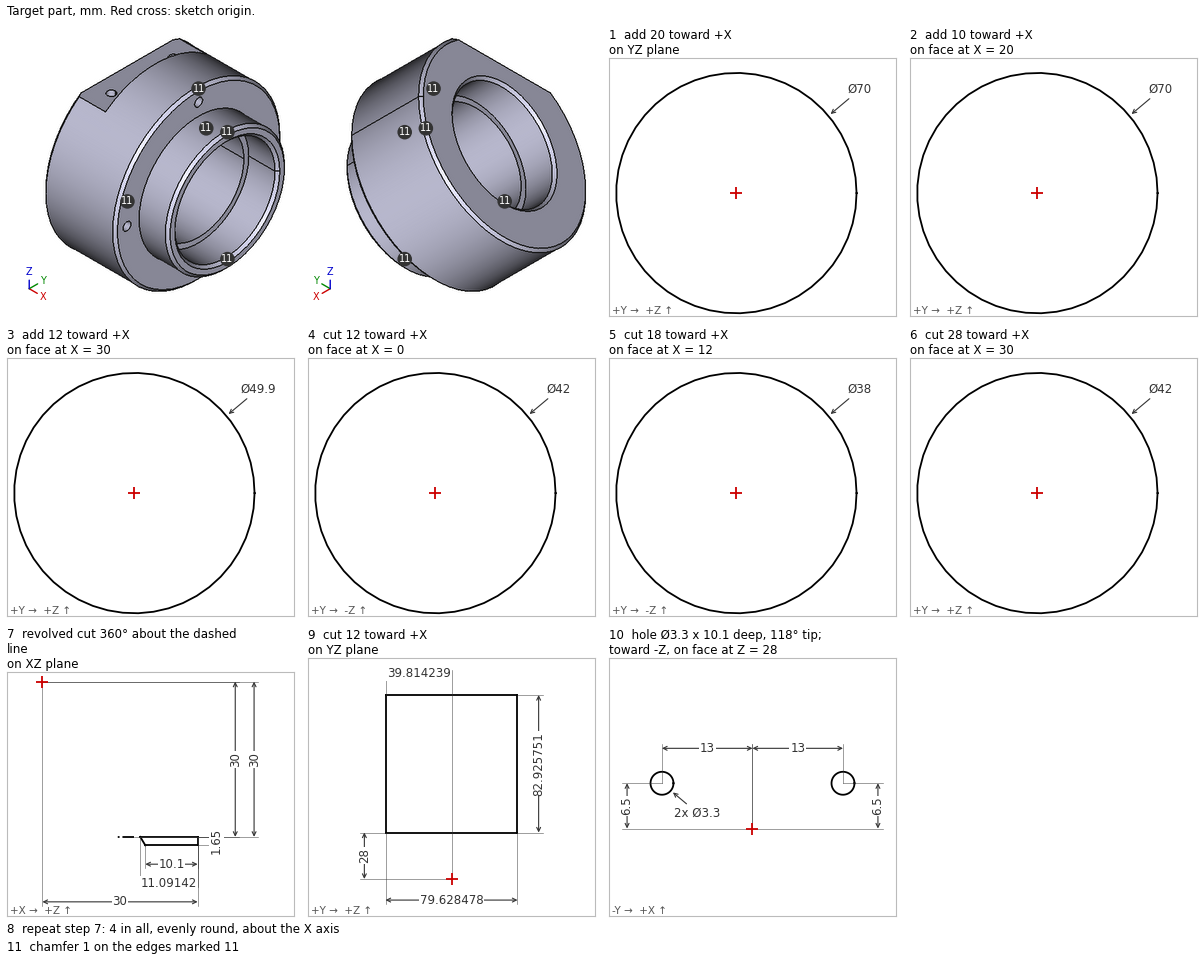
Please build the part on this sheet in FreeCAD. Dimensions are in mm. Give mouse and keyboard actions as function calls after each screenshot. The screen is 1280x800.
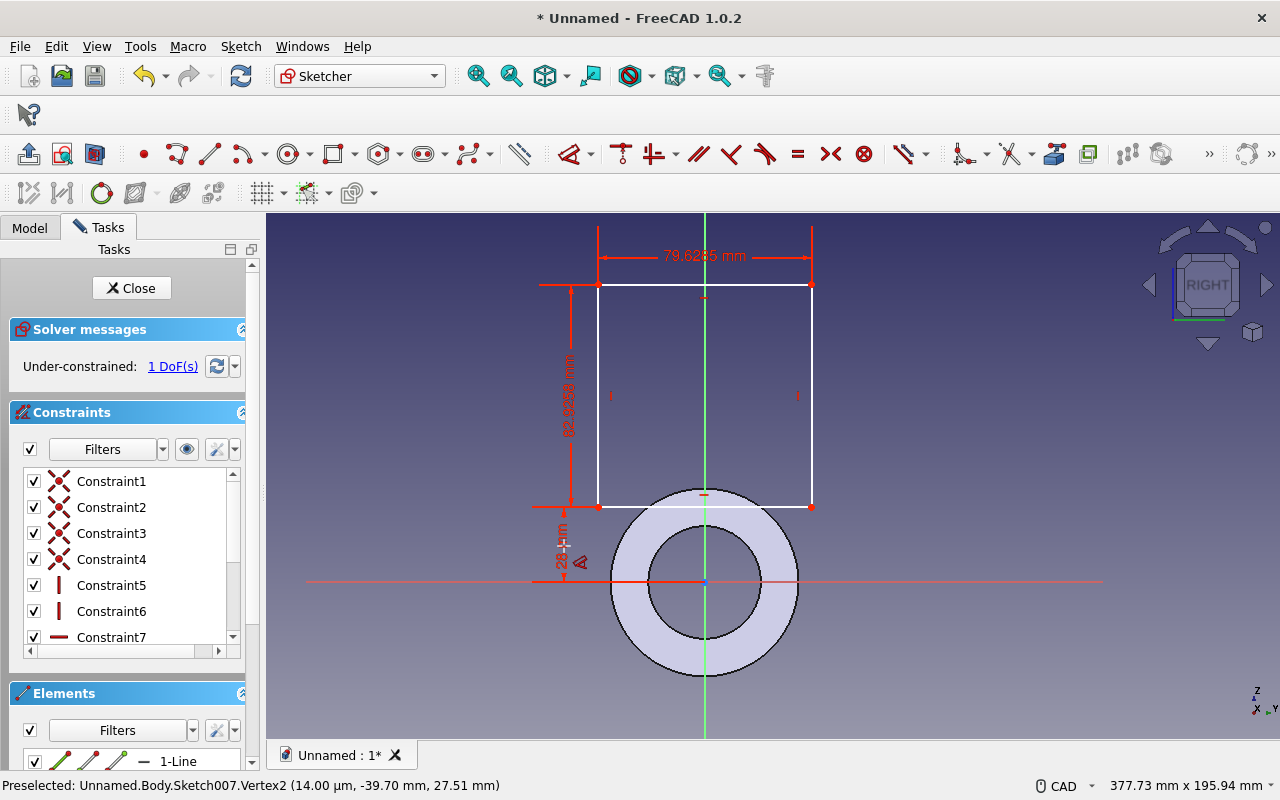
click(598, 285)
click(651, 251)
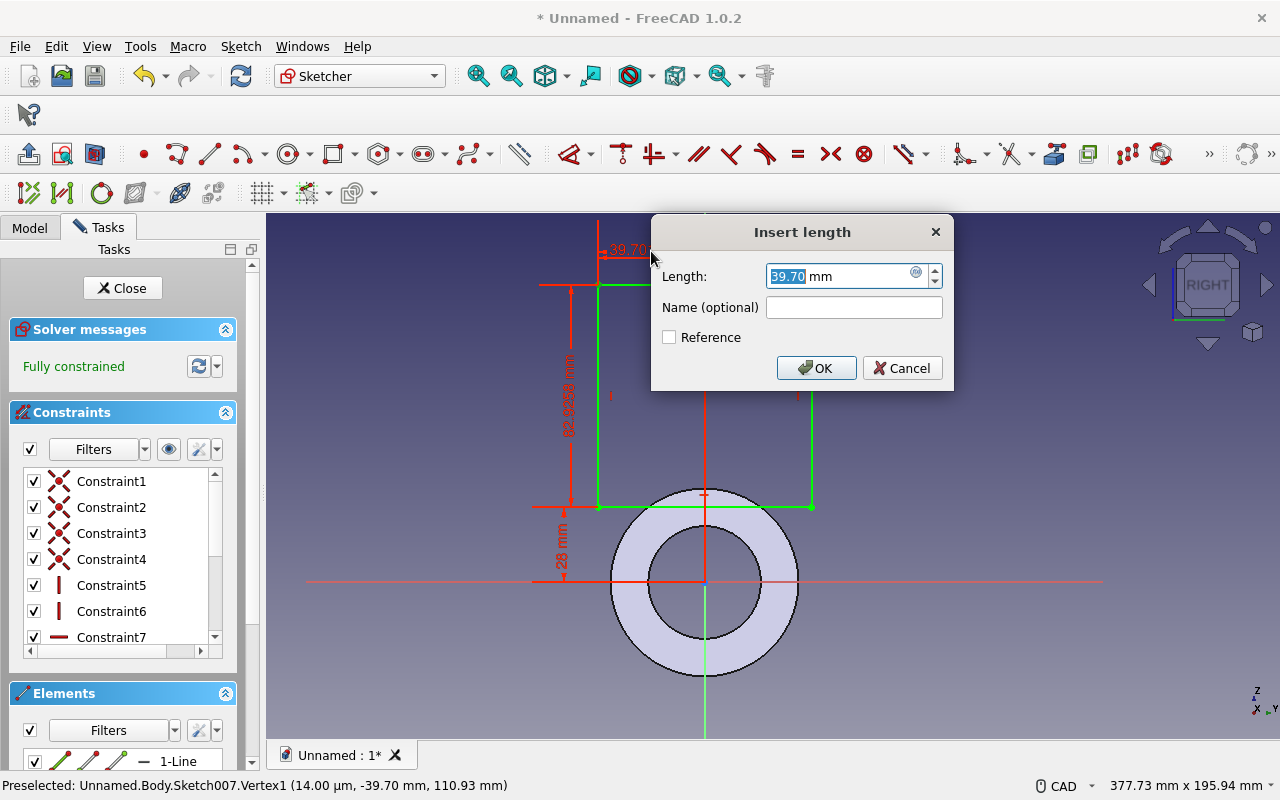
text(39.814239)
key(Return)
key(Escape)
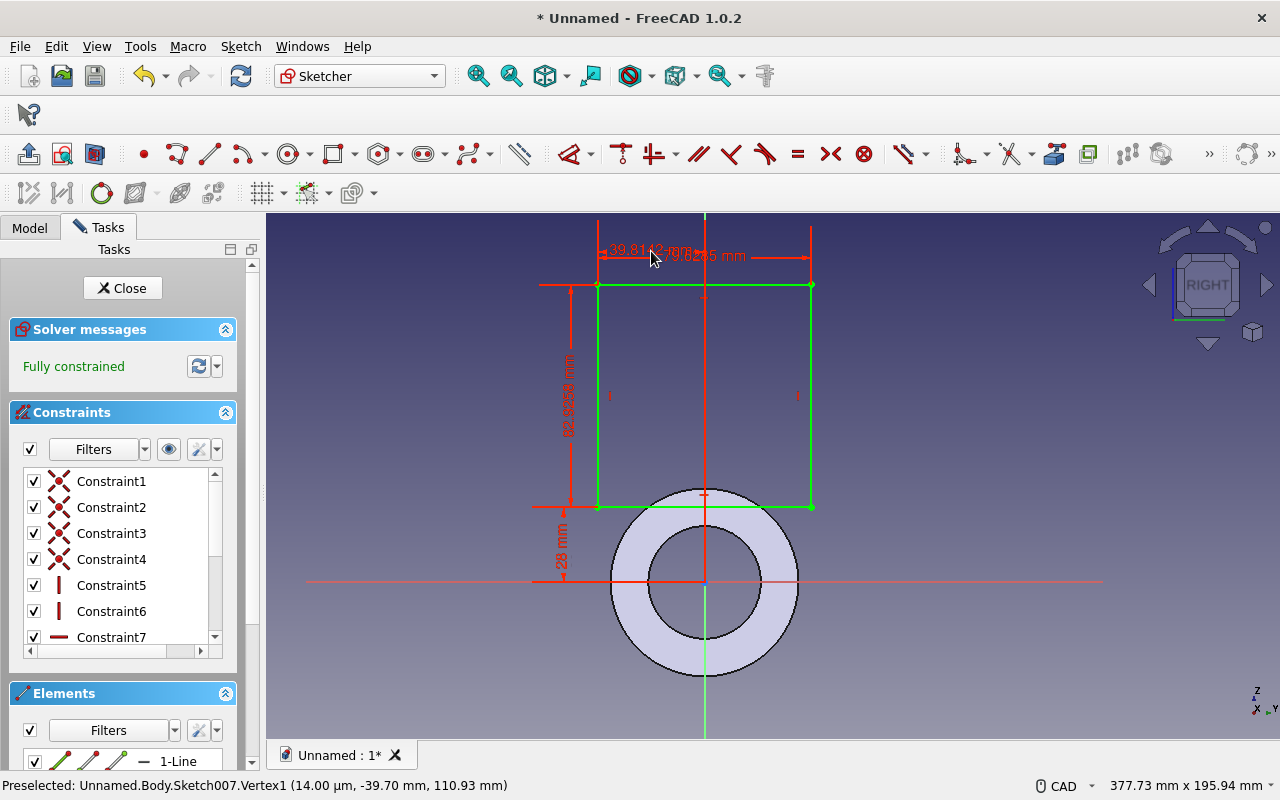
click(123, 288)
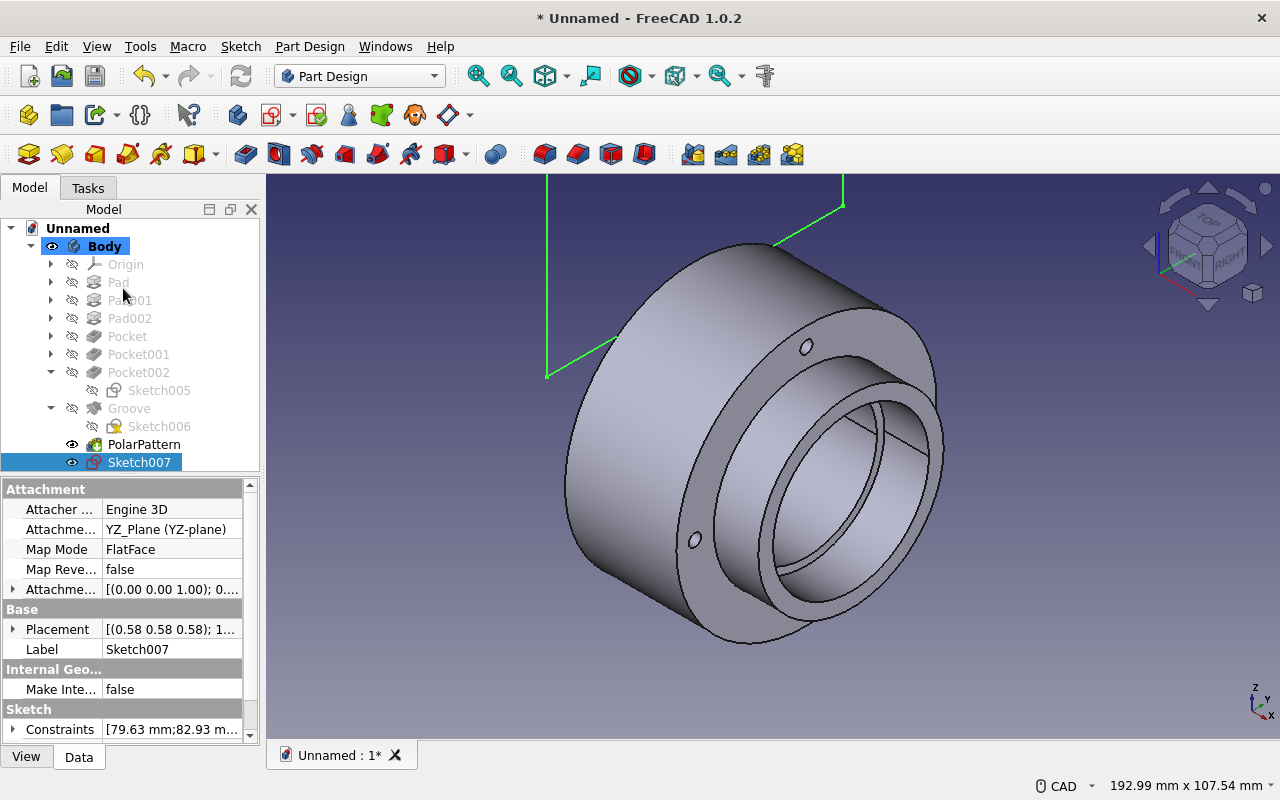
click(246, 154)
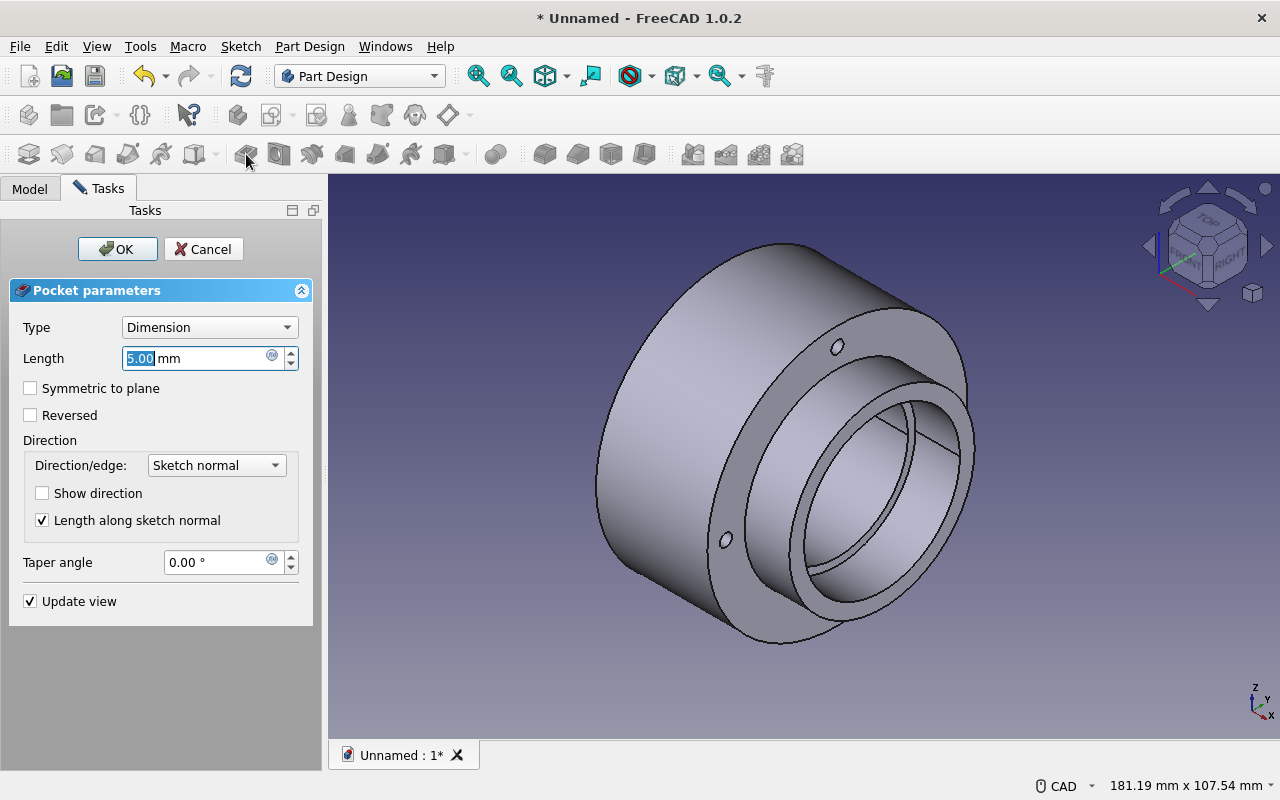
text(12)
key(Tab)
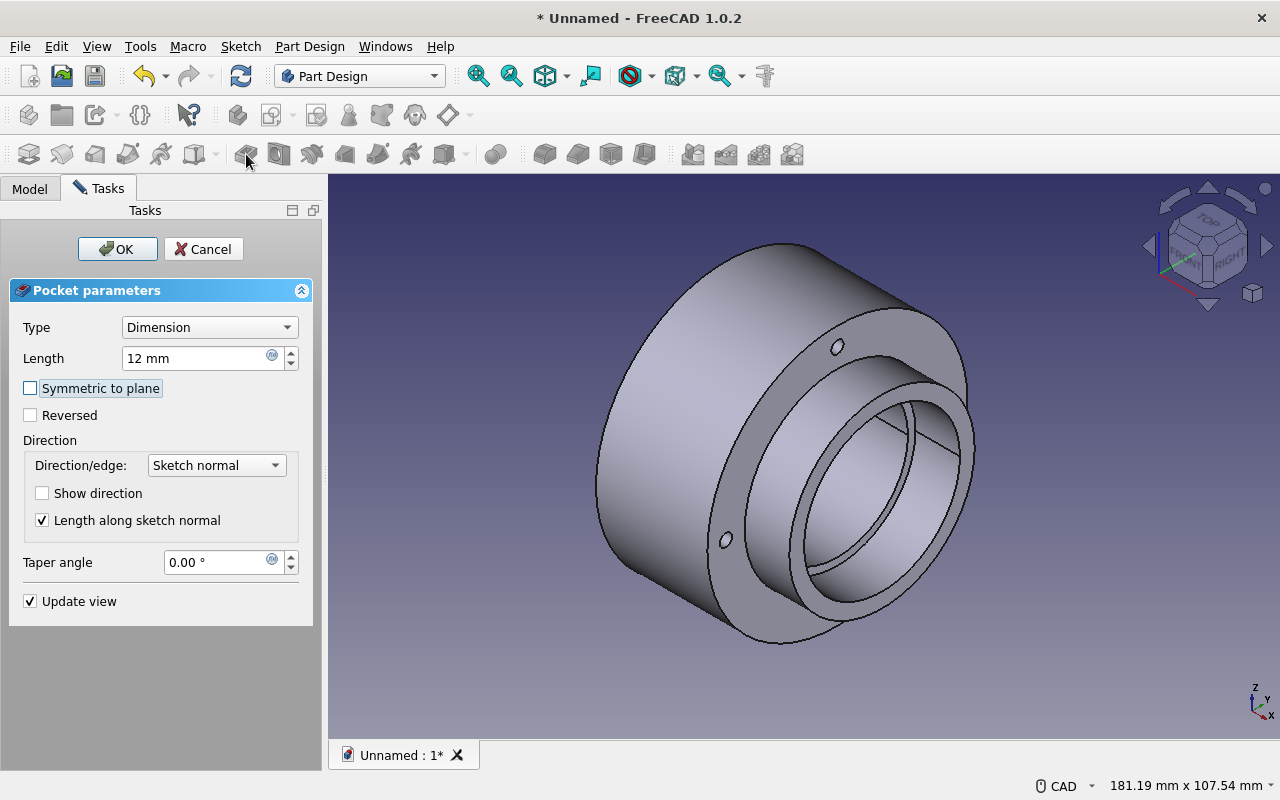
click(31, 415)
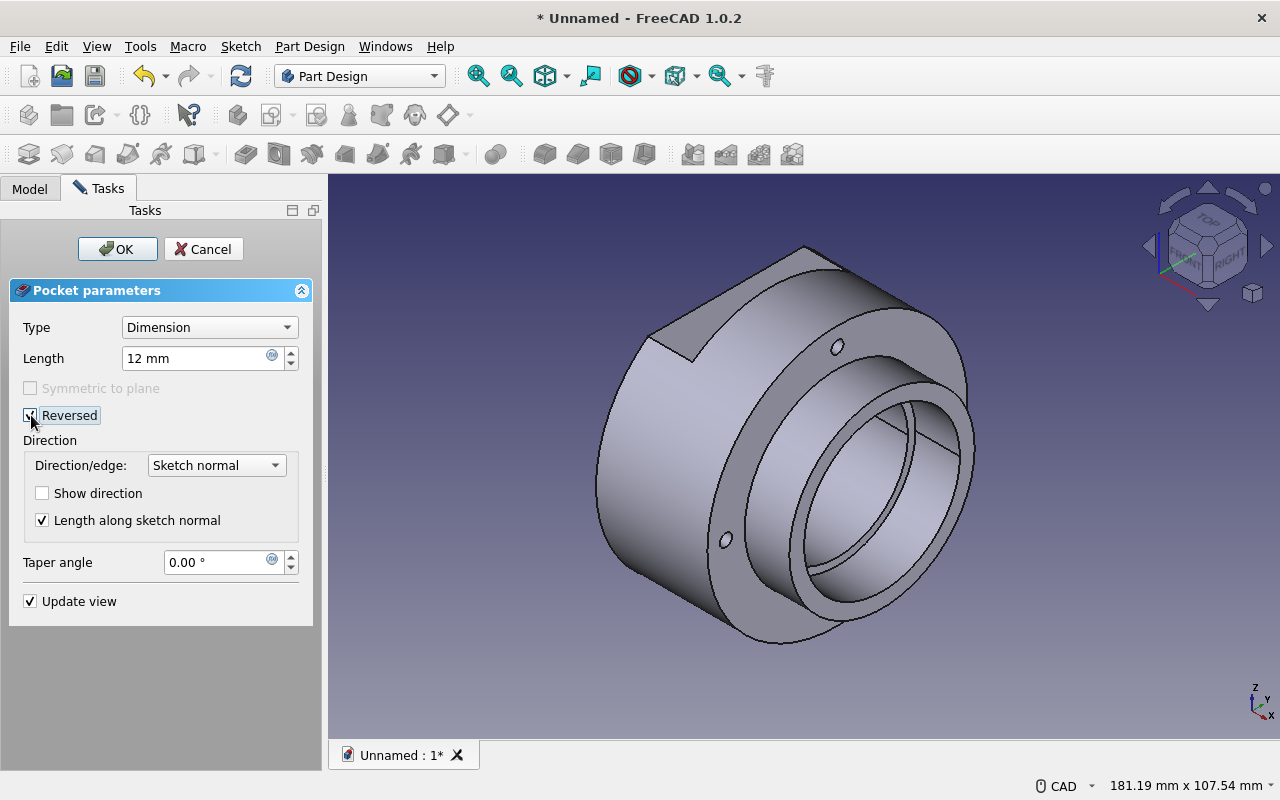
click(118, 249)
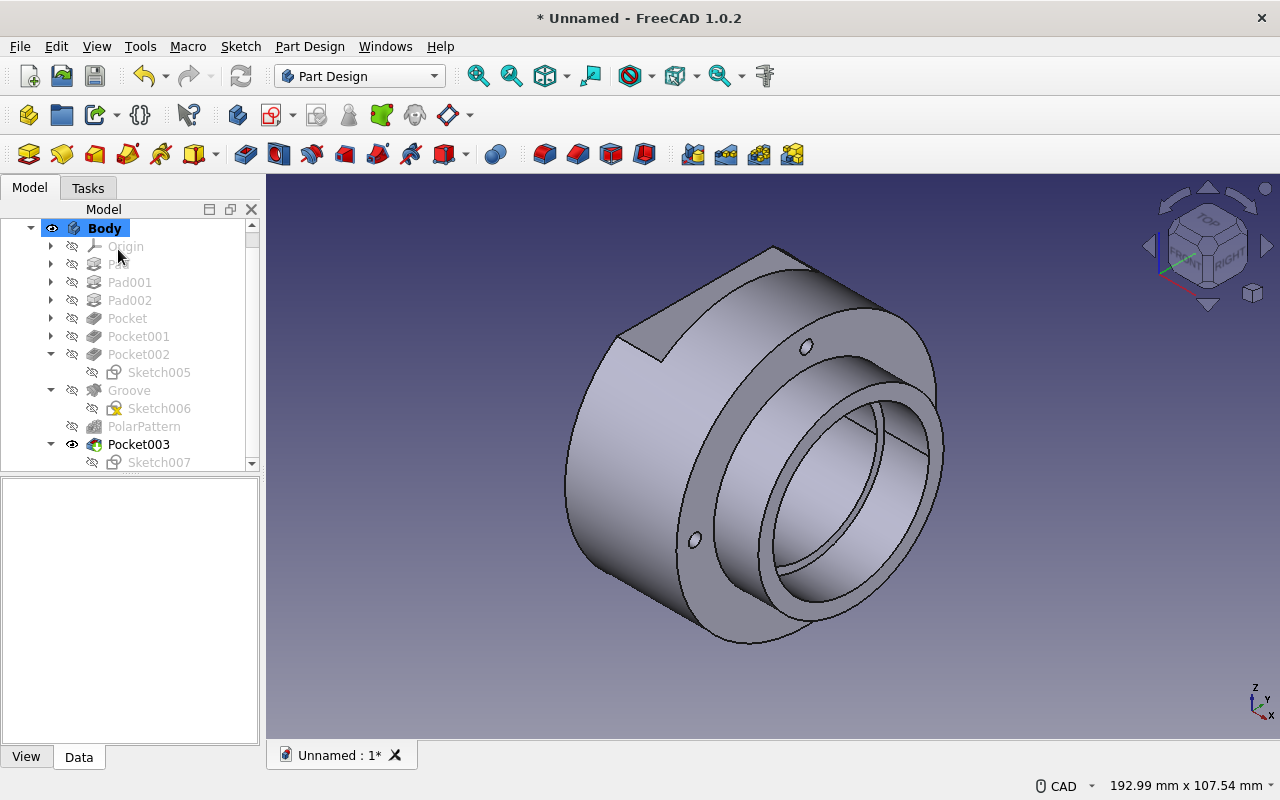
click(673, 329)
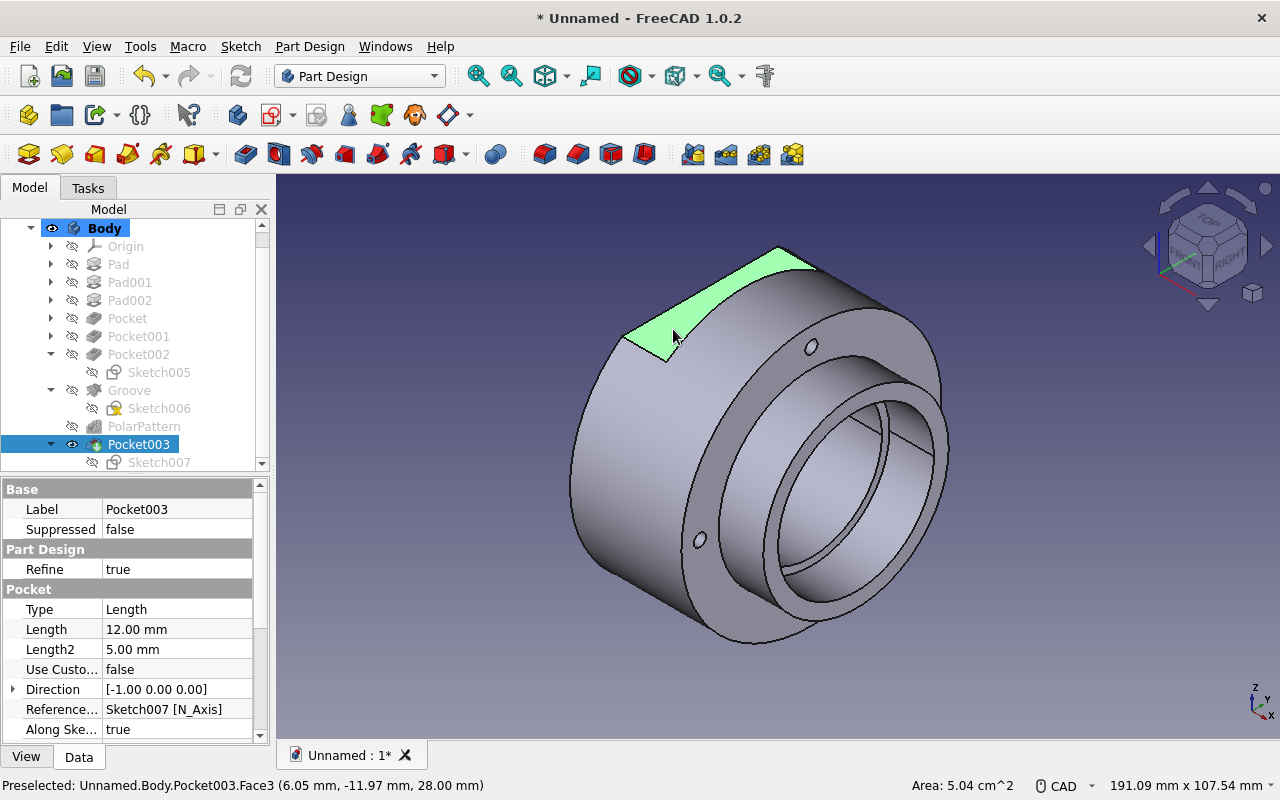
click(270, 116)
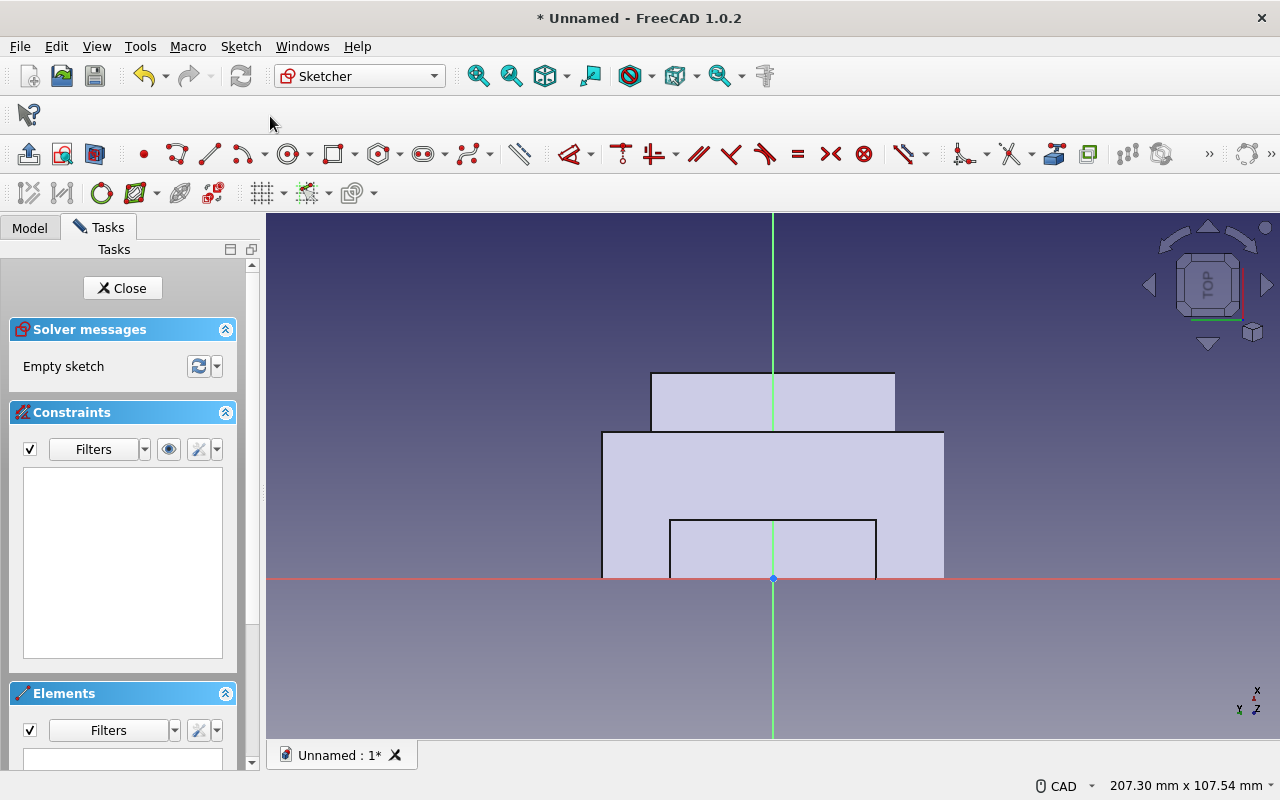
click(95, 154)